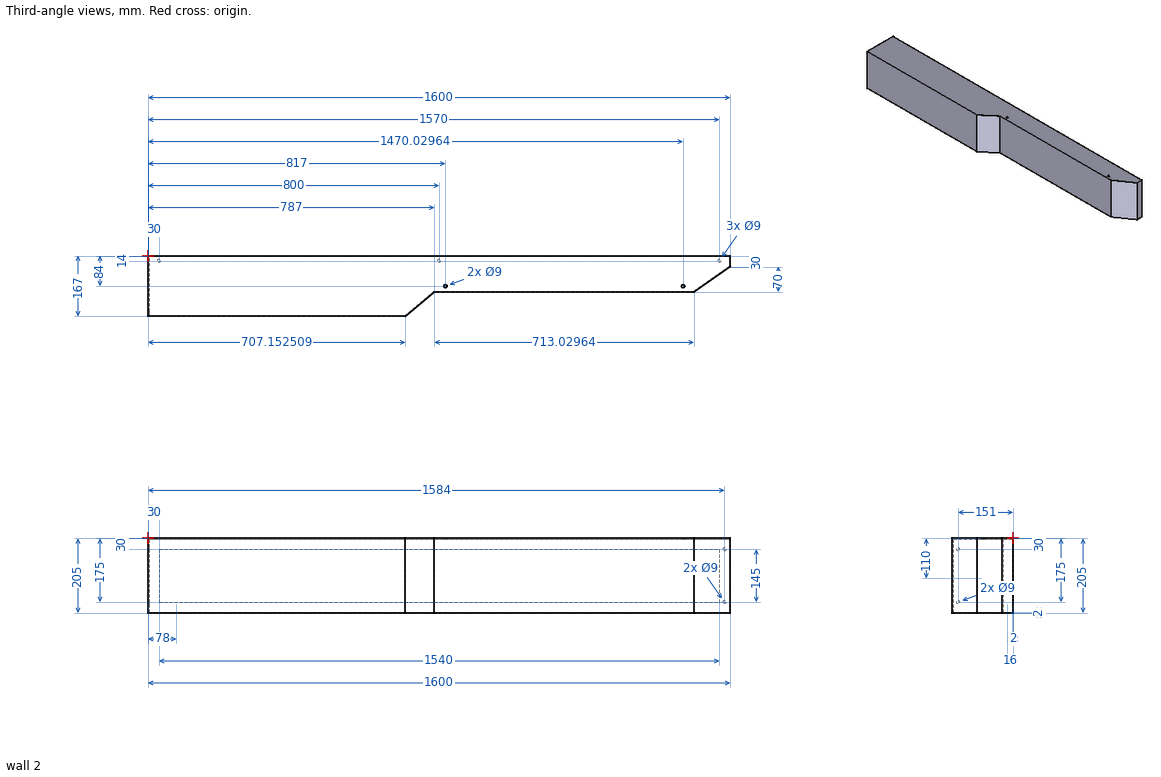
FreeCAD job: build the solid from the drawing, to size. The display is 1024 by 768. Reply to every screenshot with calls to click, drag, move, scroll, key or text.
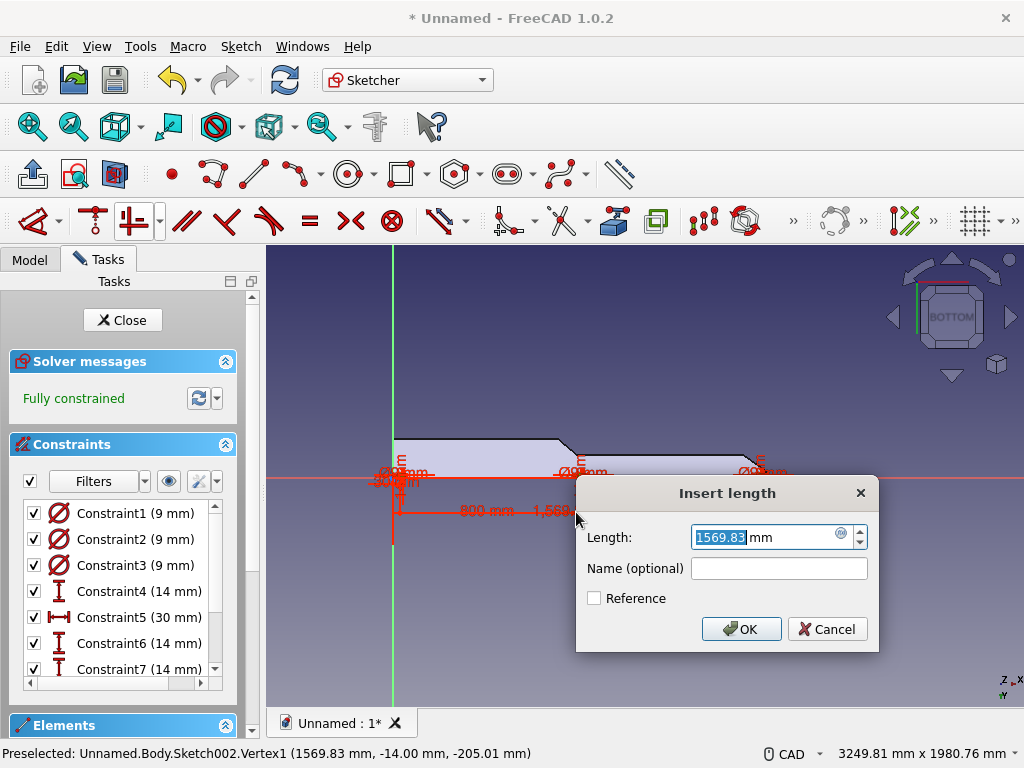
text(1570)
key(Return)
key(Escape)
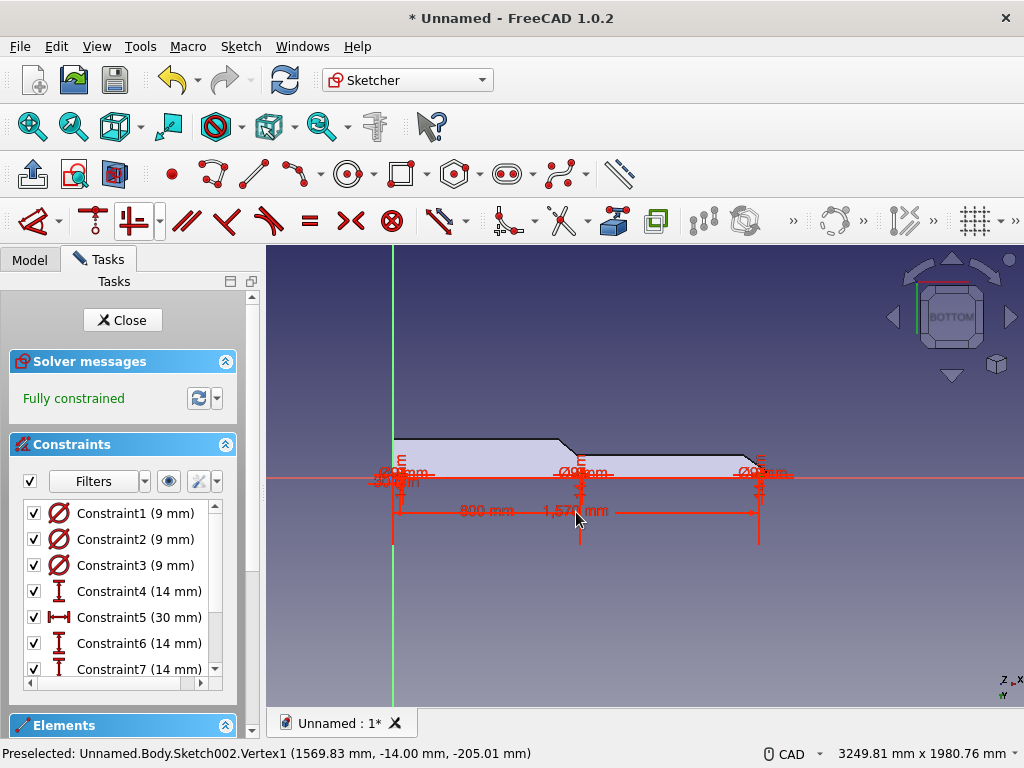
click(123, 320)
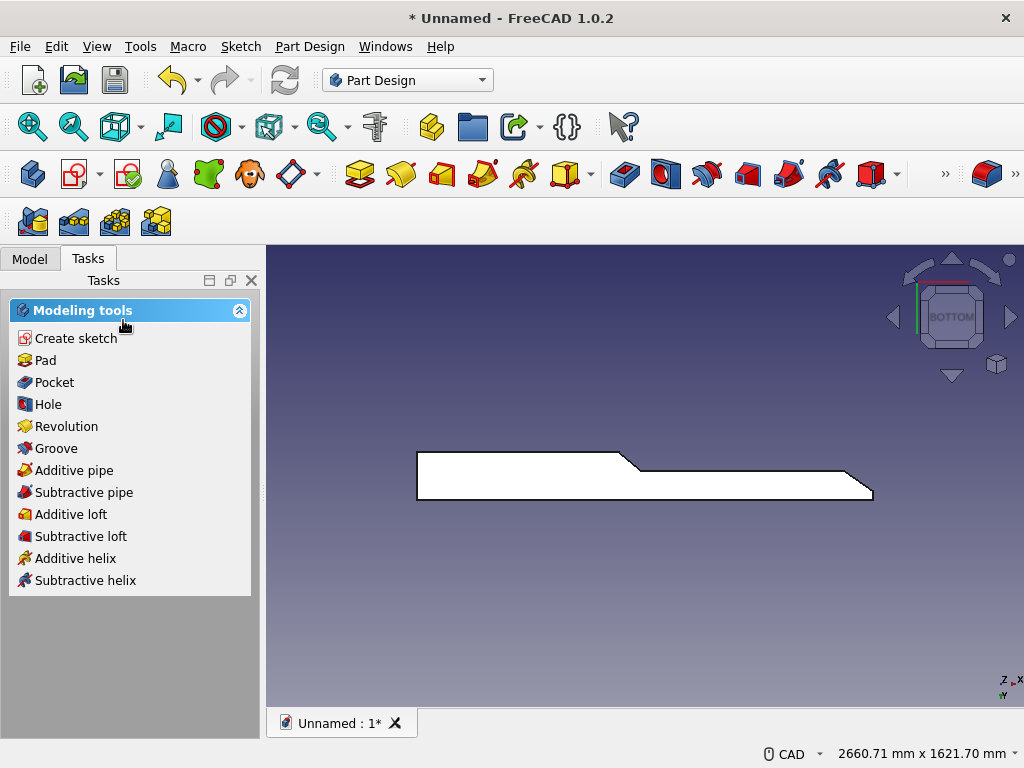
click(625, 174)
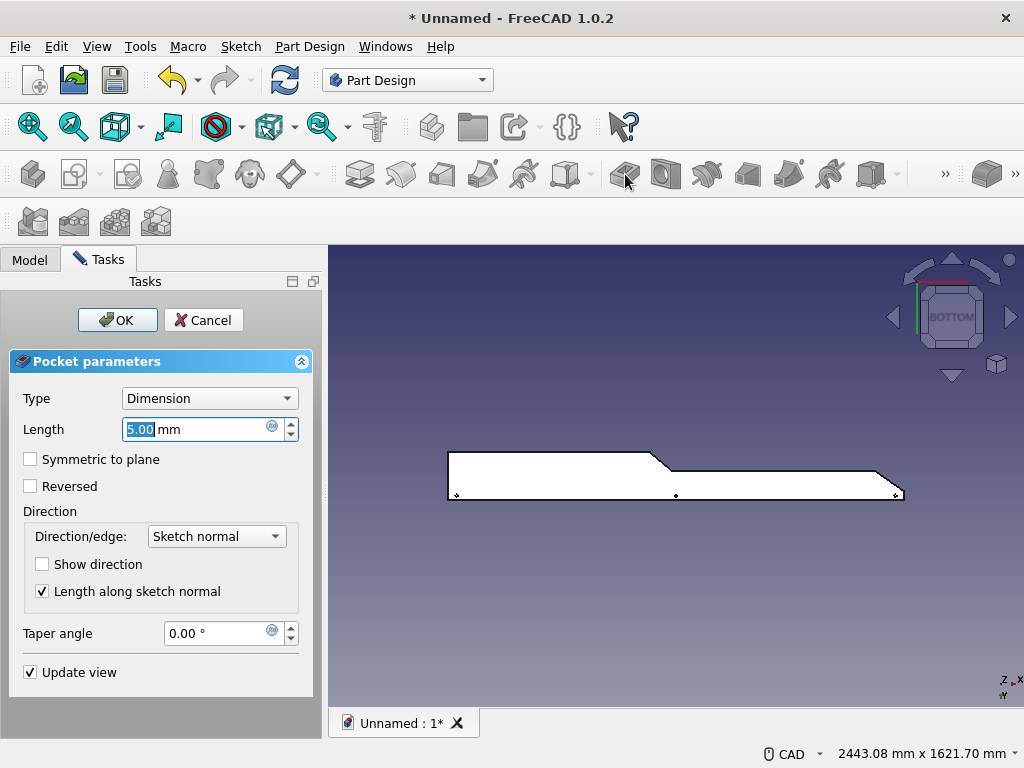
text(2)
key(Tab)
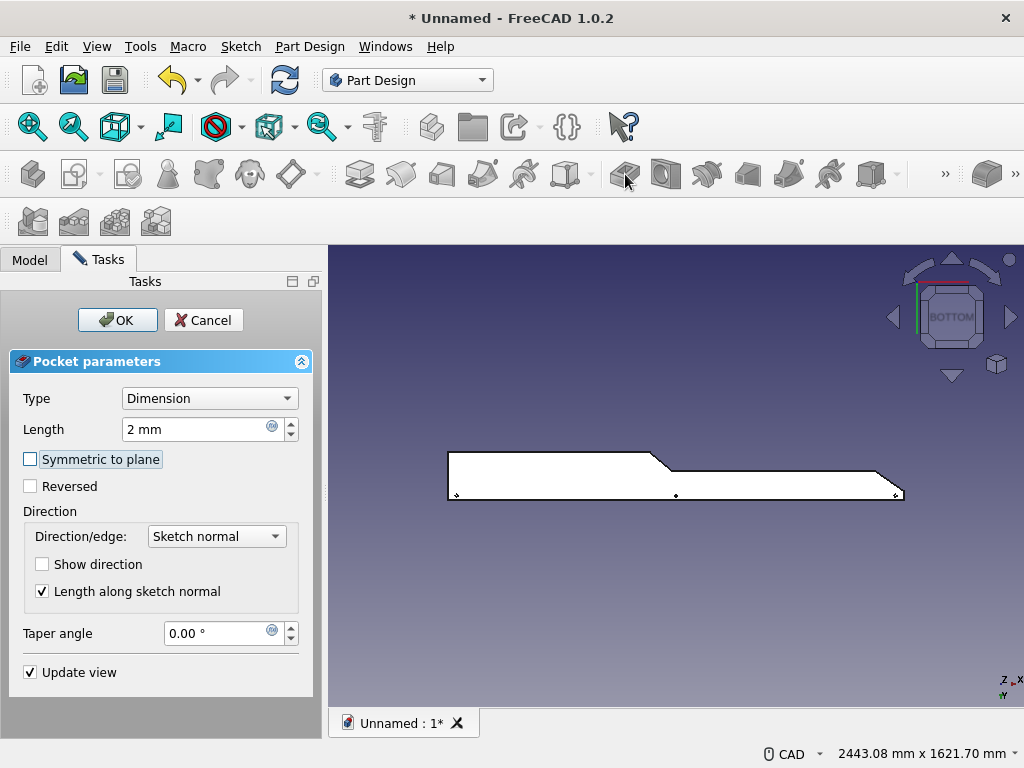
click(118, 320)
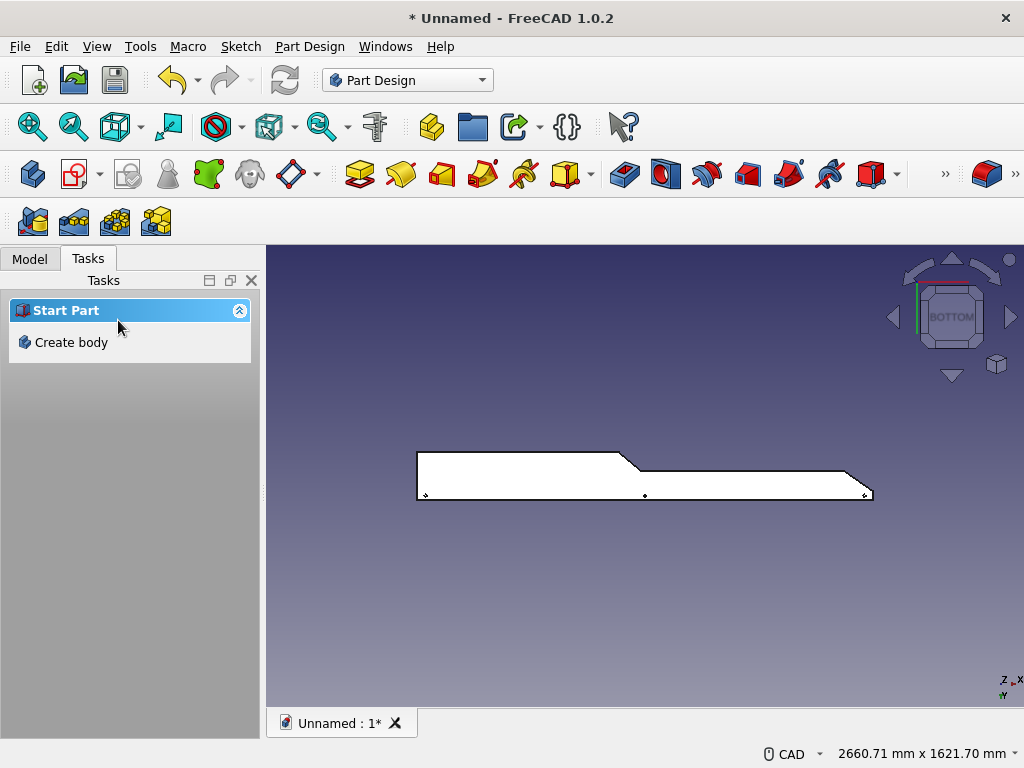
key(6)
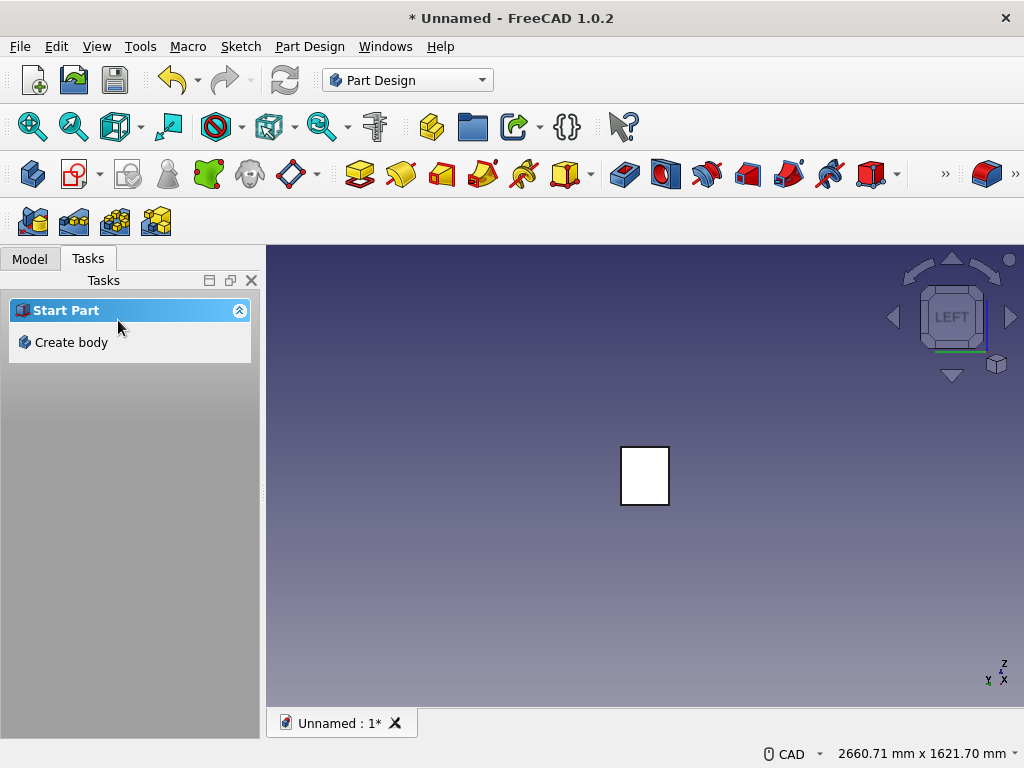
click(33, 128)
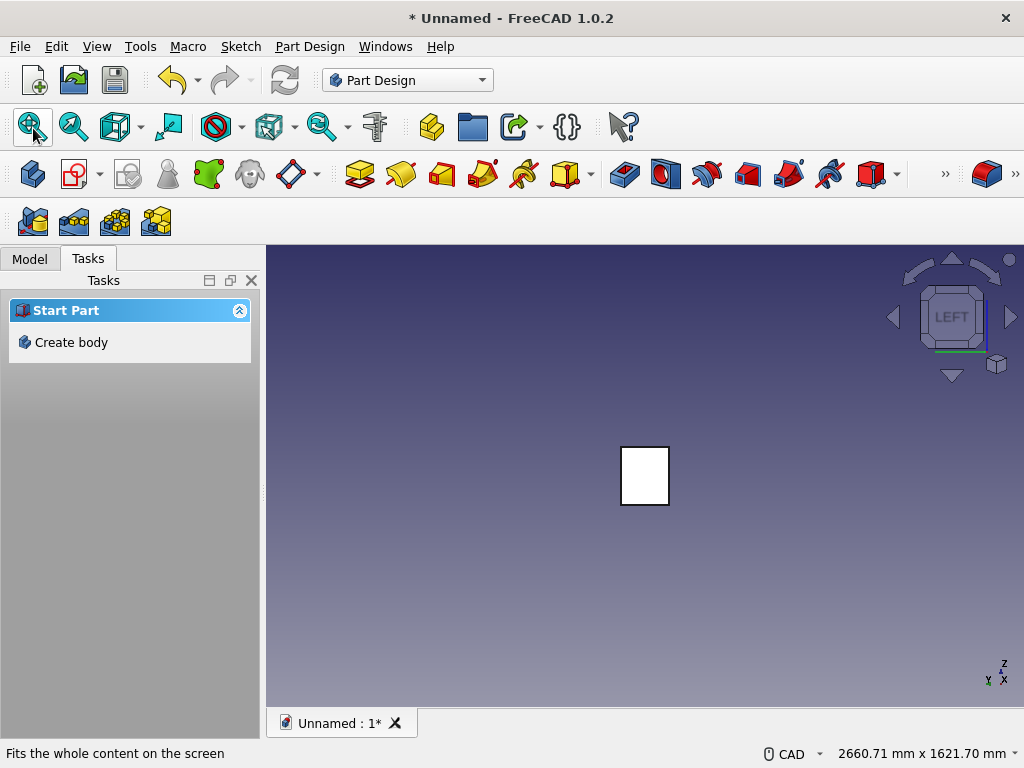
click(645, 475)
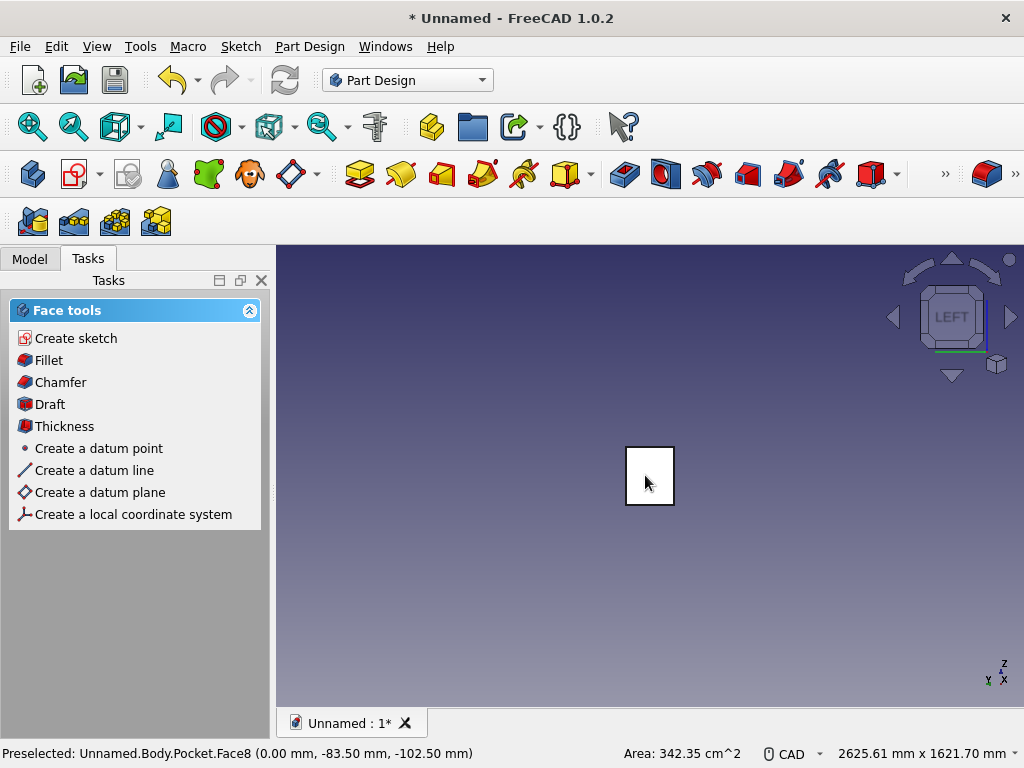
click(74, 174)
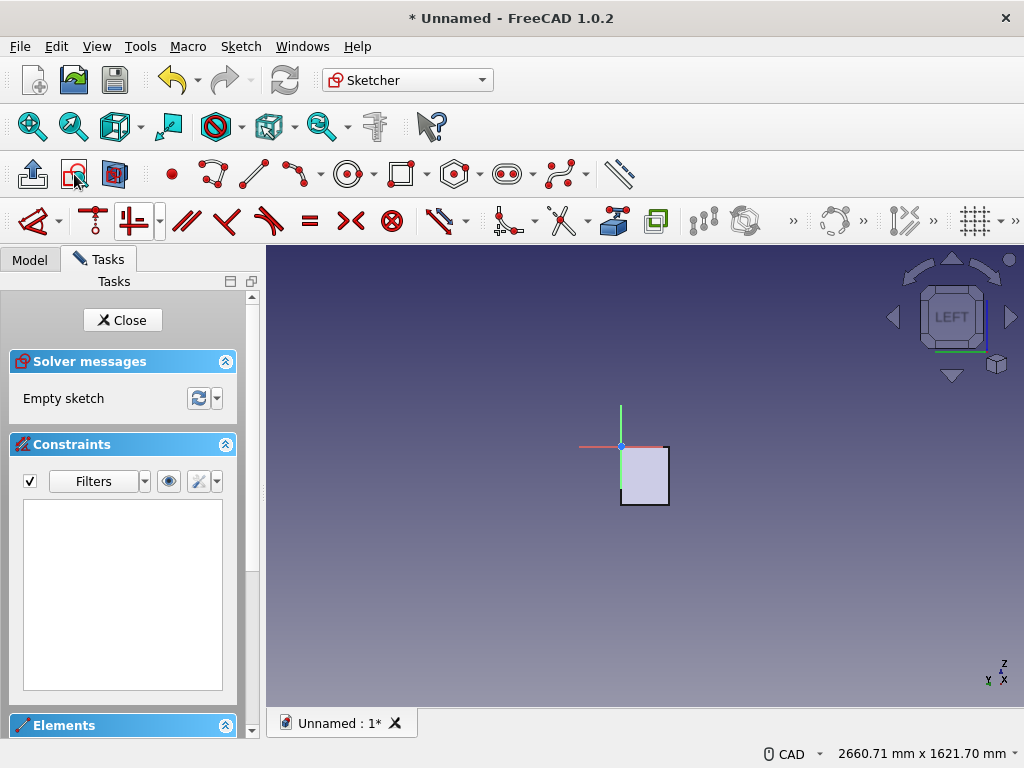
scroll(657, 472, up, 9)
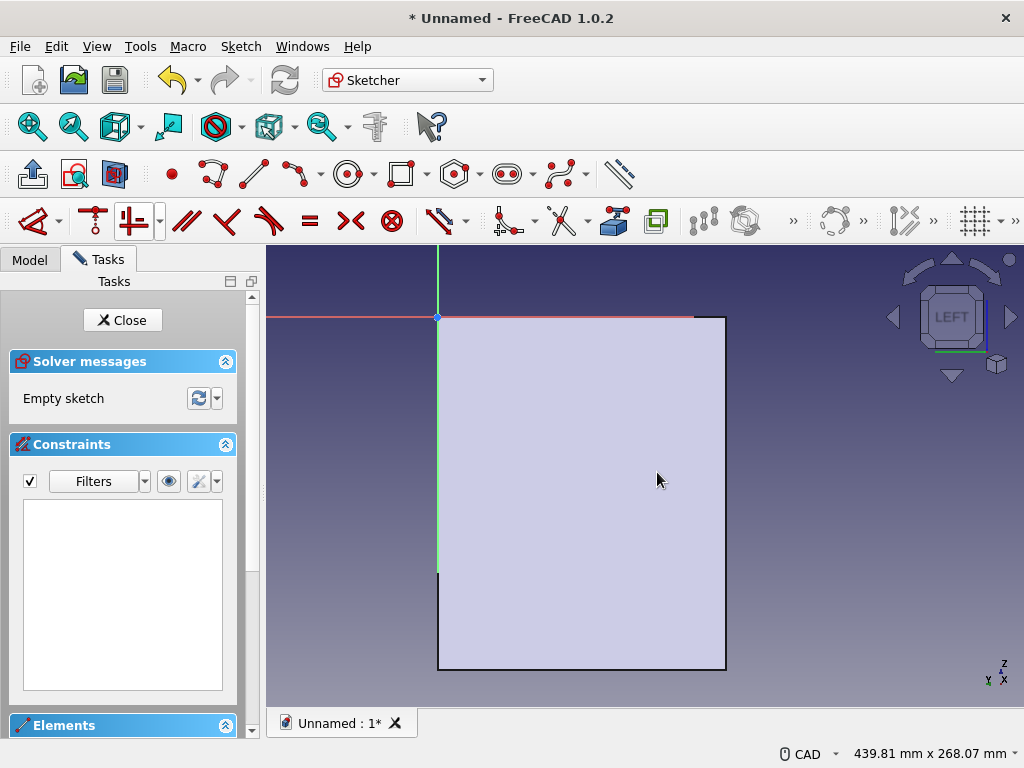
key(g)
key(c)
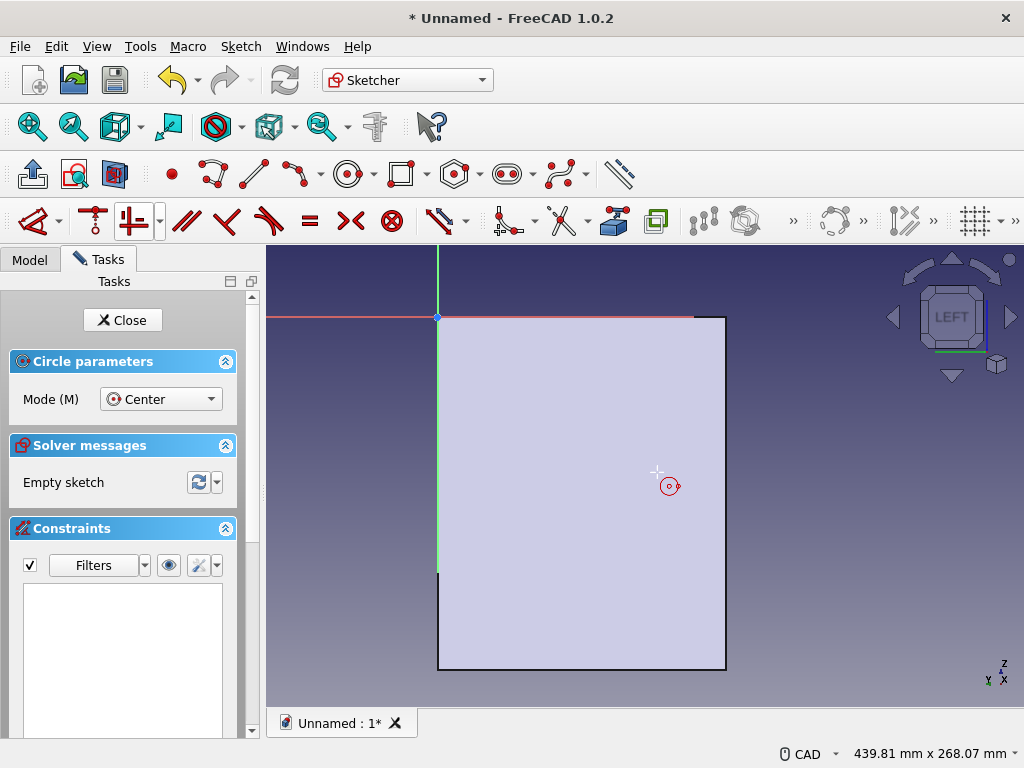
scroll(698, 619, up, 6)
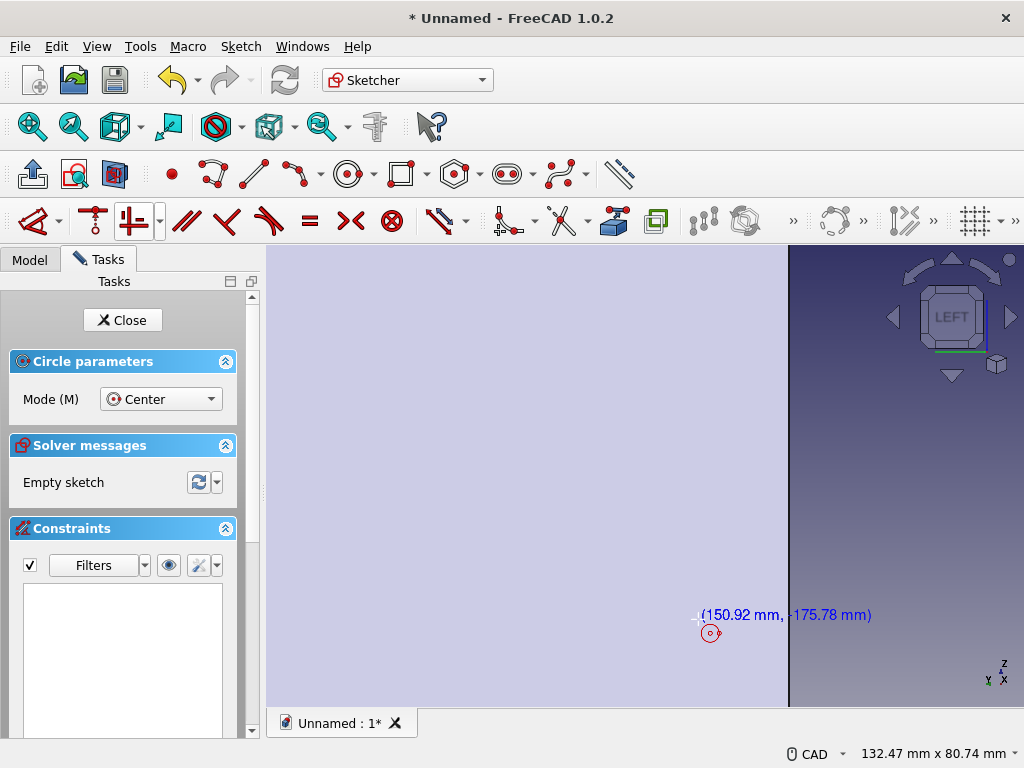
click(697, 616)
move(715, 598)